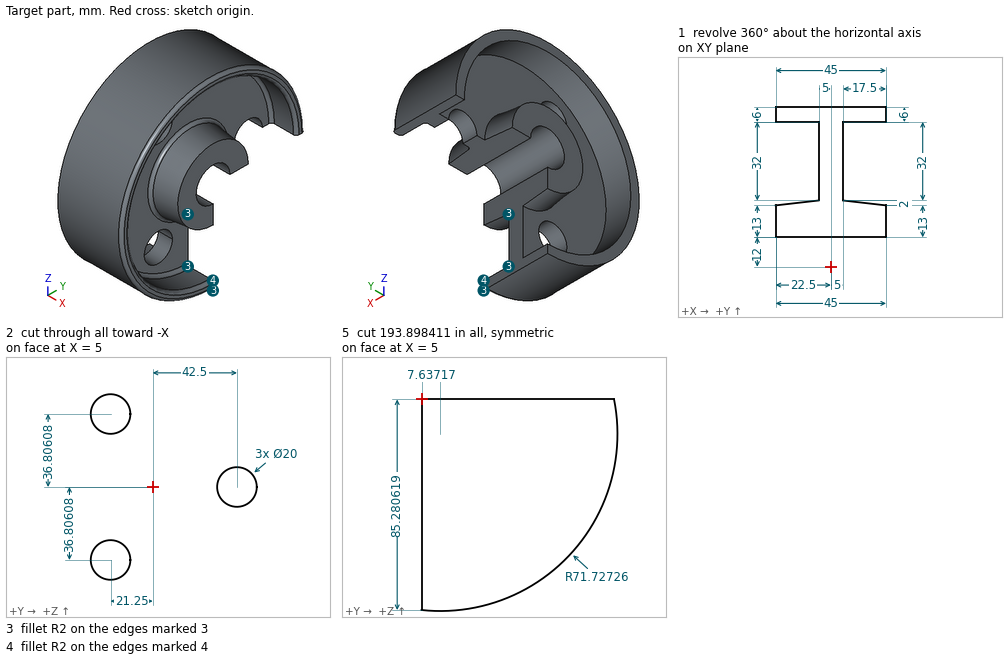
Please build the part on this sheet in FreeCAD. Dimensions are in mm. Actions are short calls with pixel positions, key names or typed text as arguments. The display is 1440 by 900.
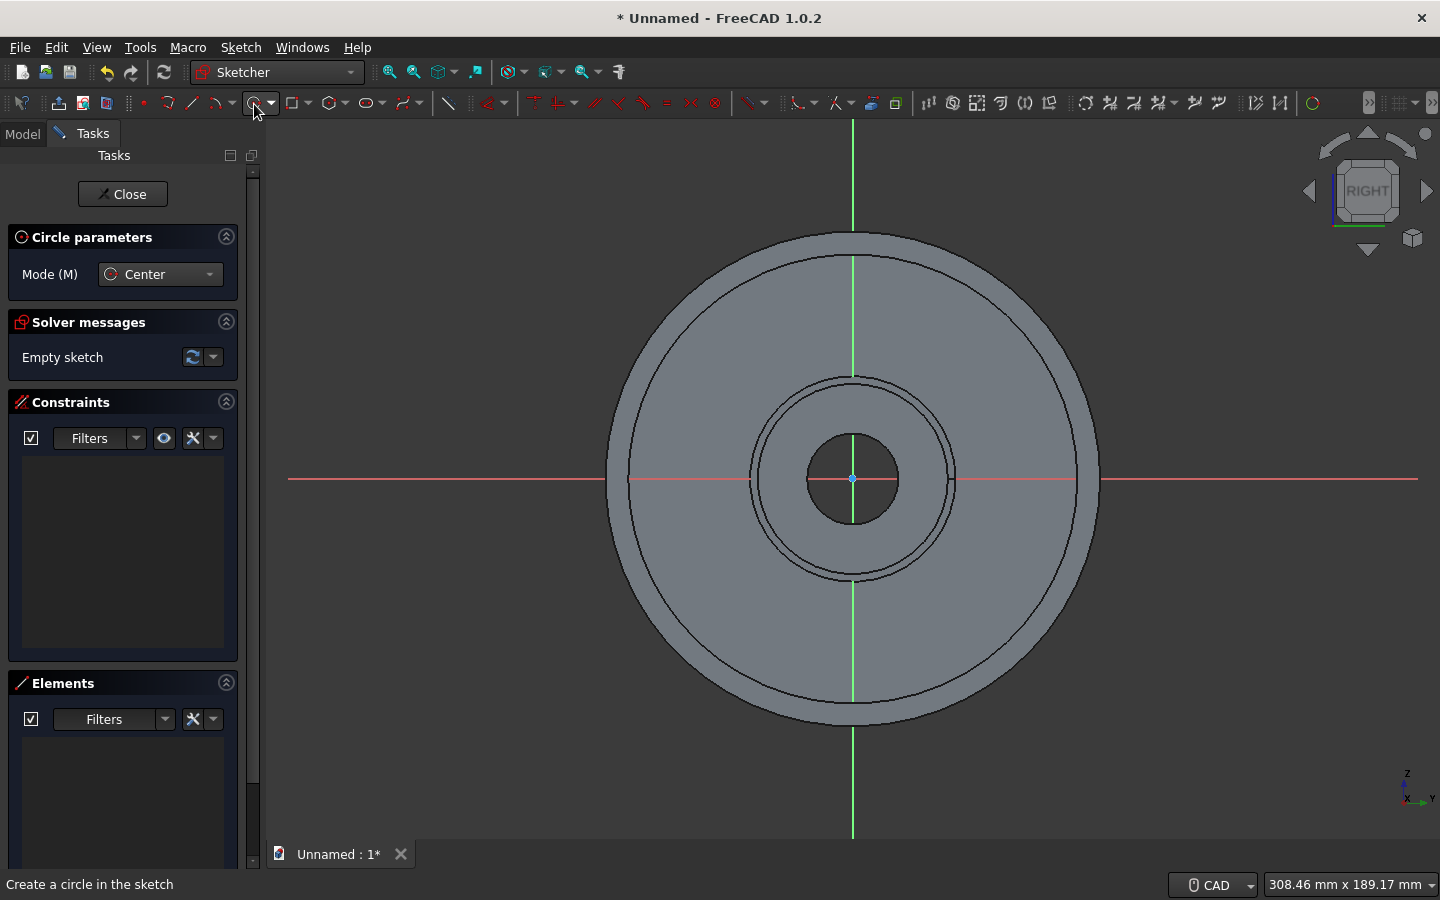
click(1015, 479)
move(1041, 452)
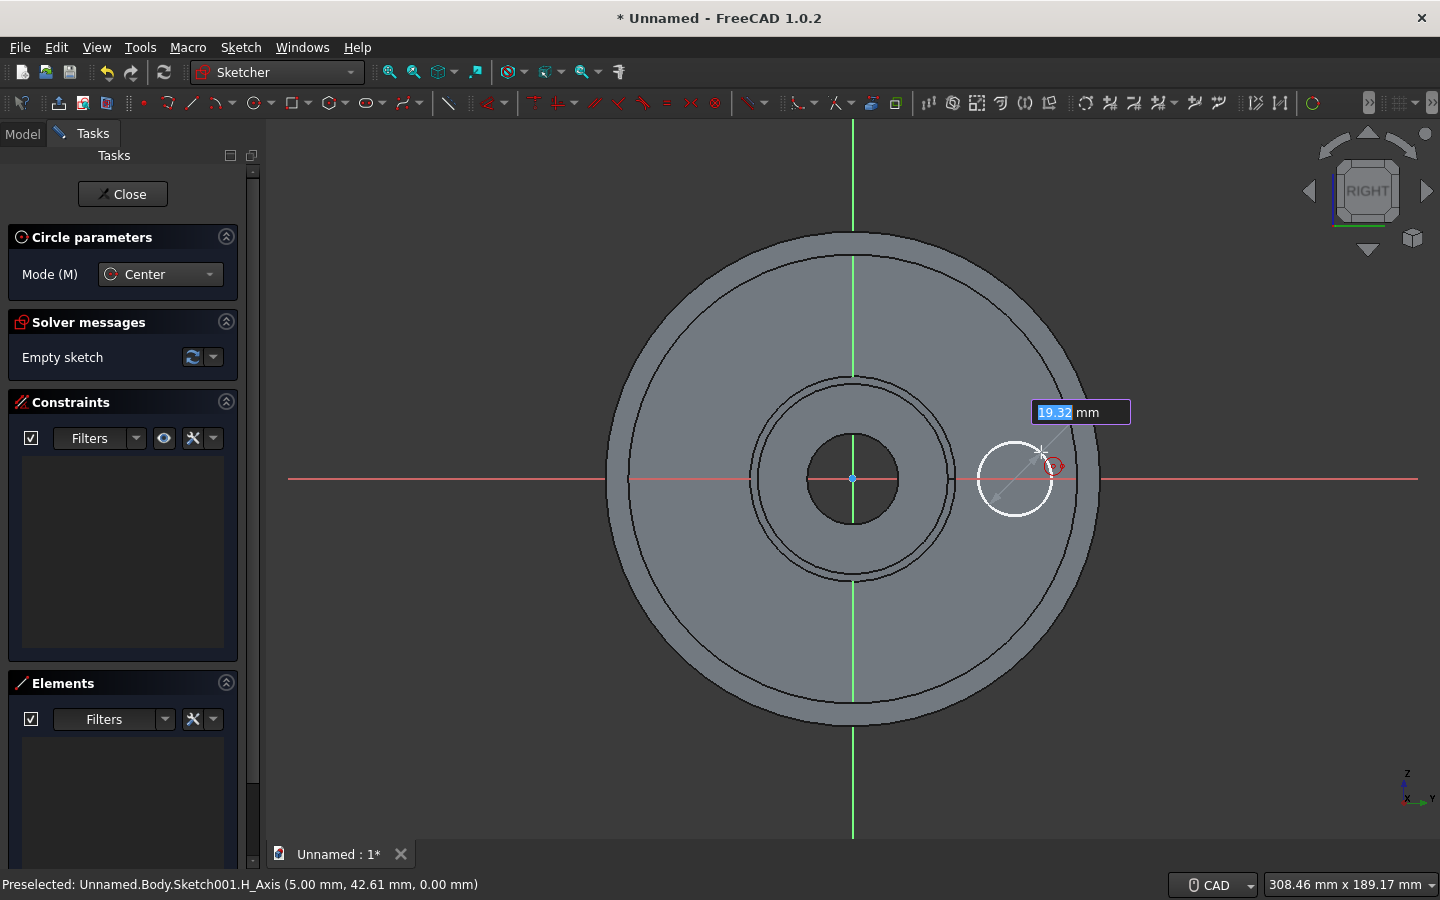
text(20)
key(Return)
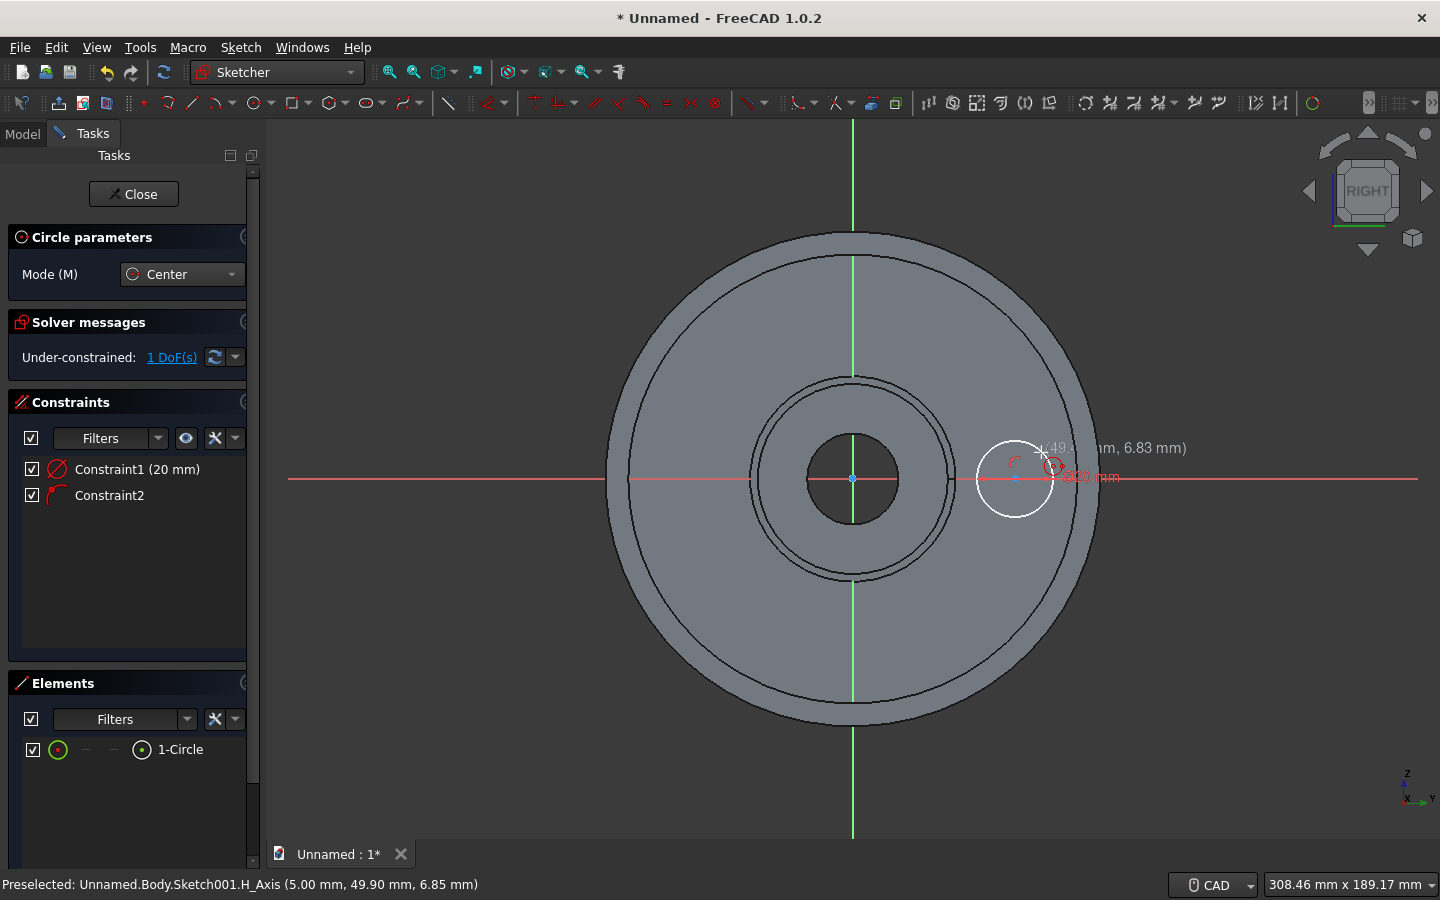
click(772, 619)
move(799, 592)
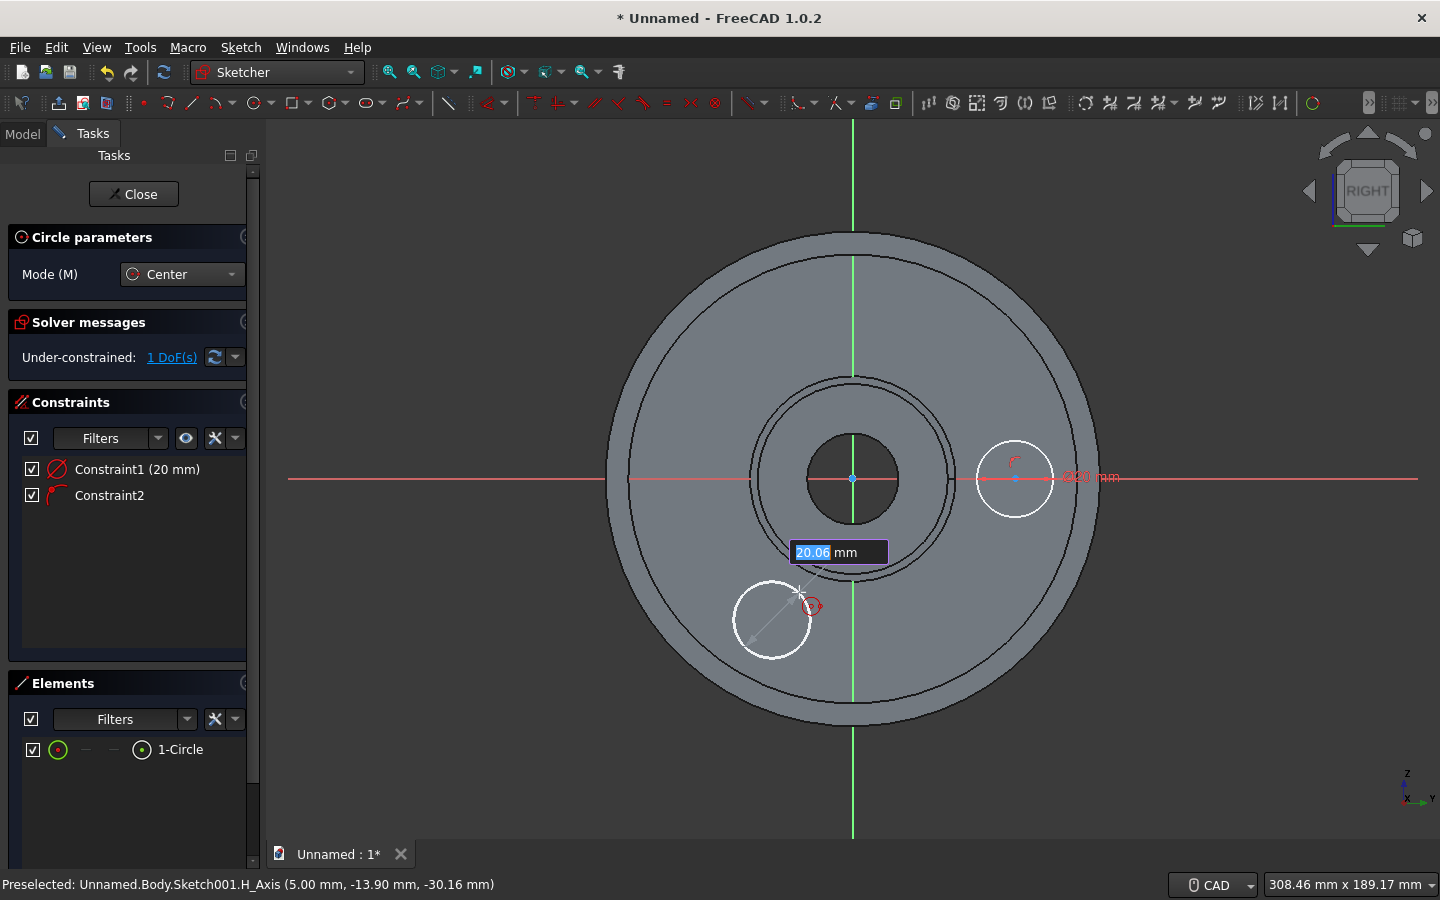
text(20)
key(Return)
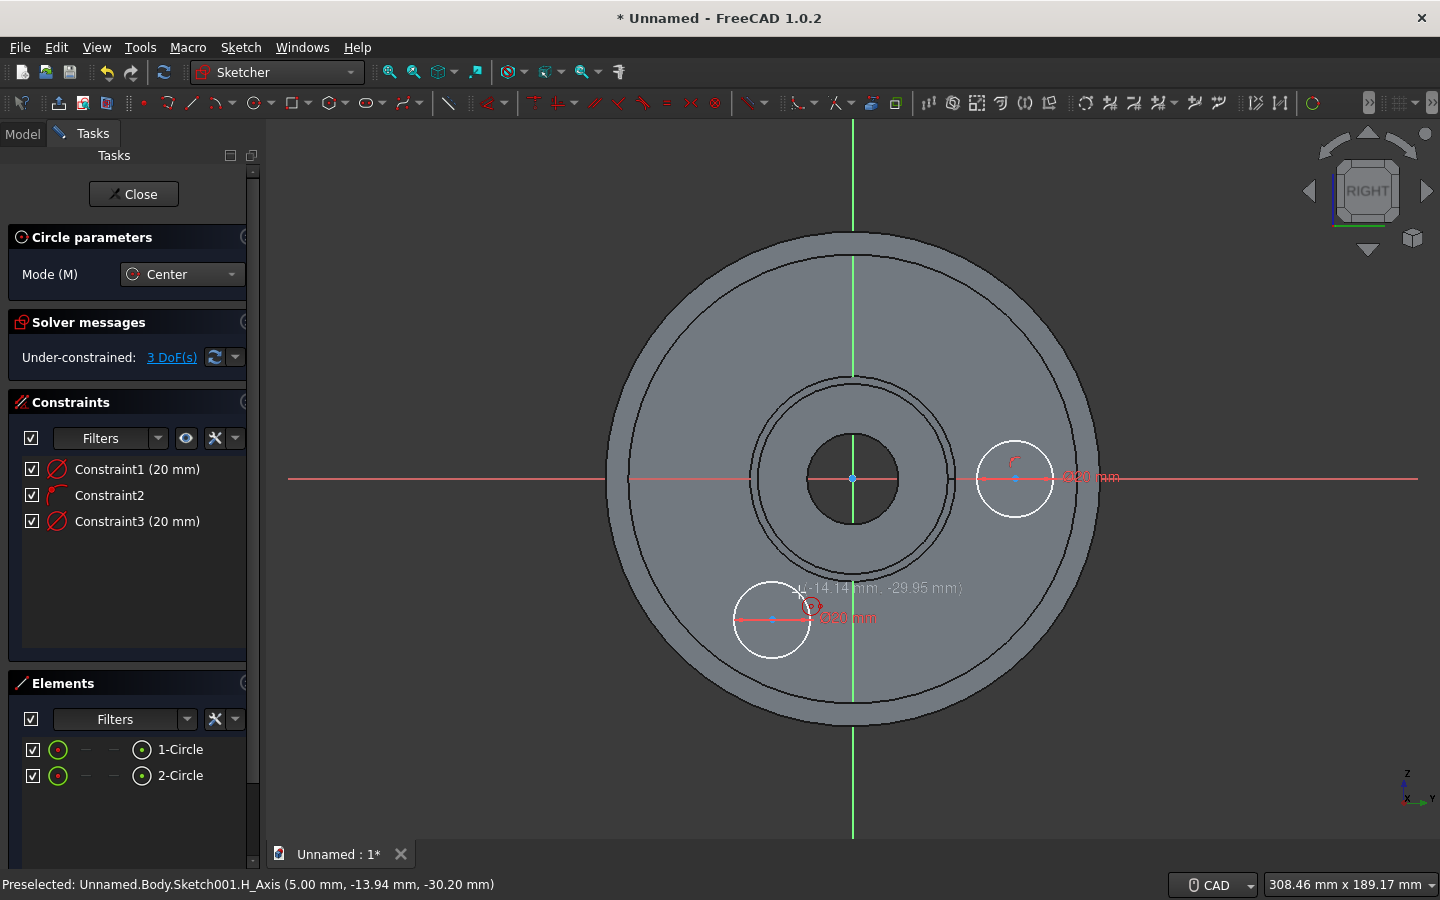
click(772, 339)
move(799, 312)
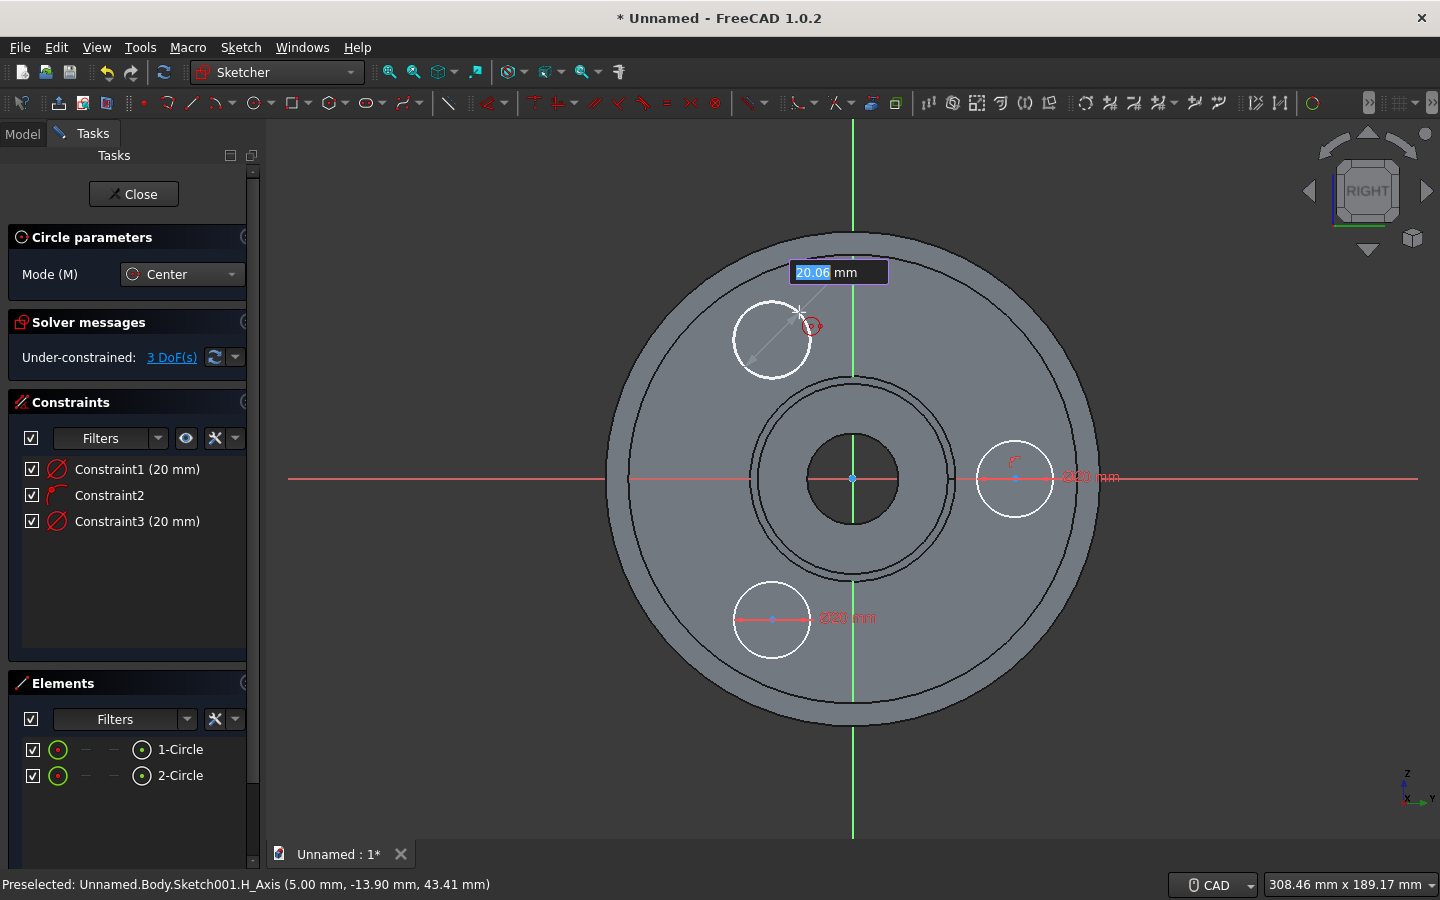
text(20)
key(Return)
key(Escape)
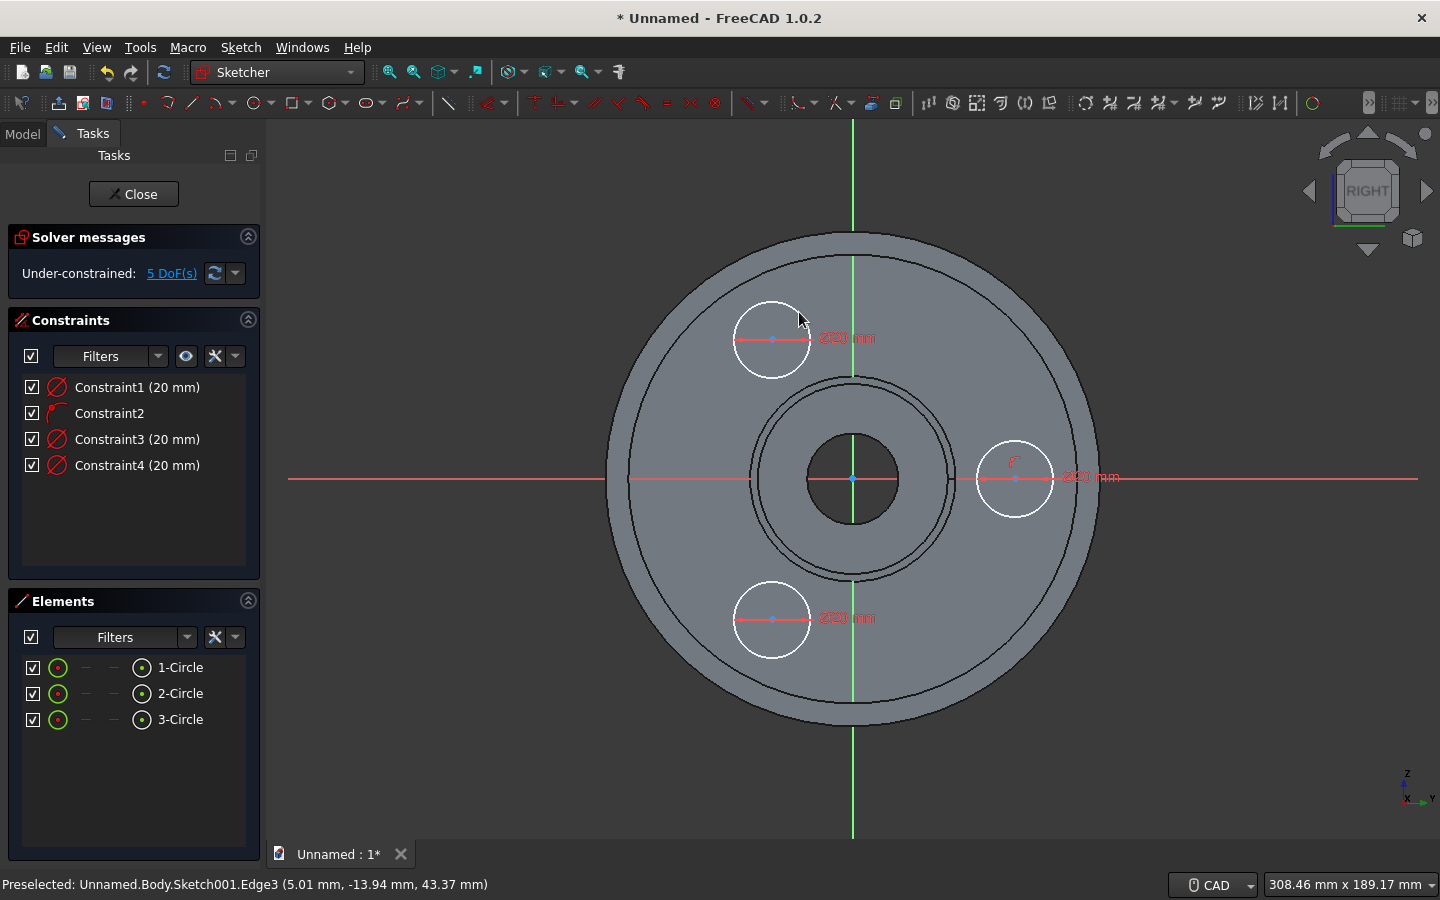
click(772, 620)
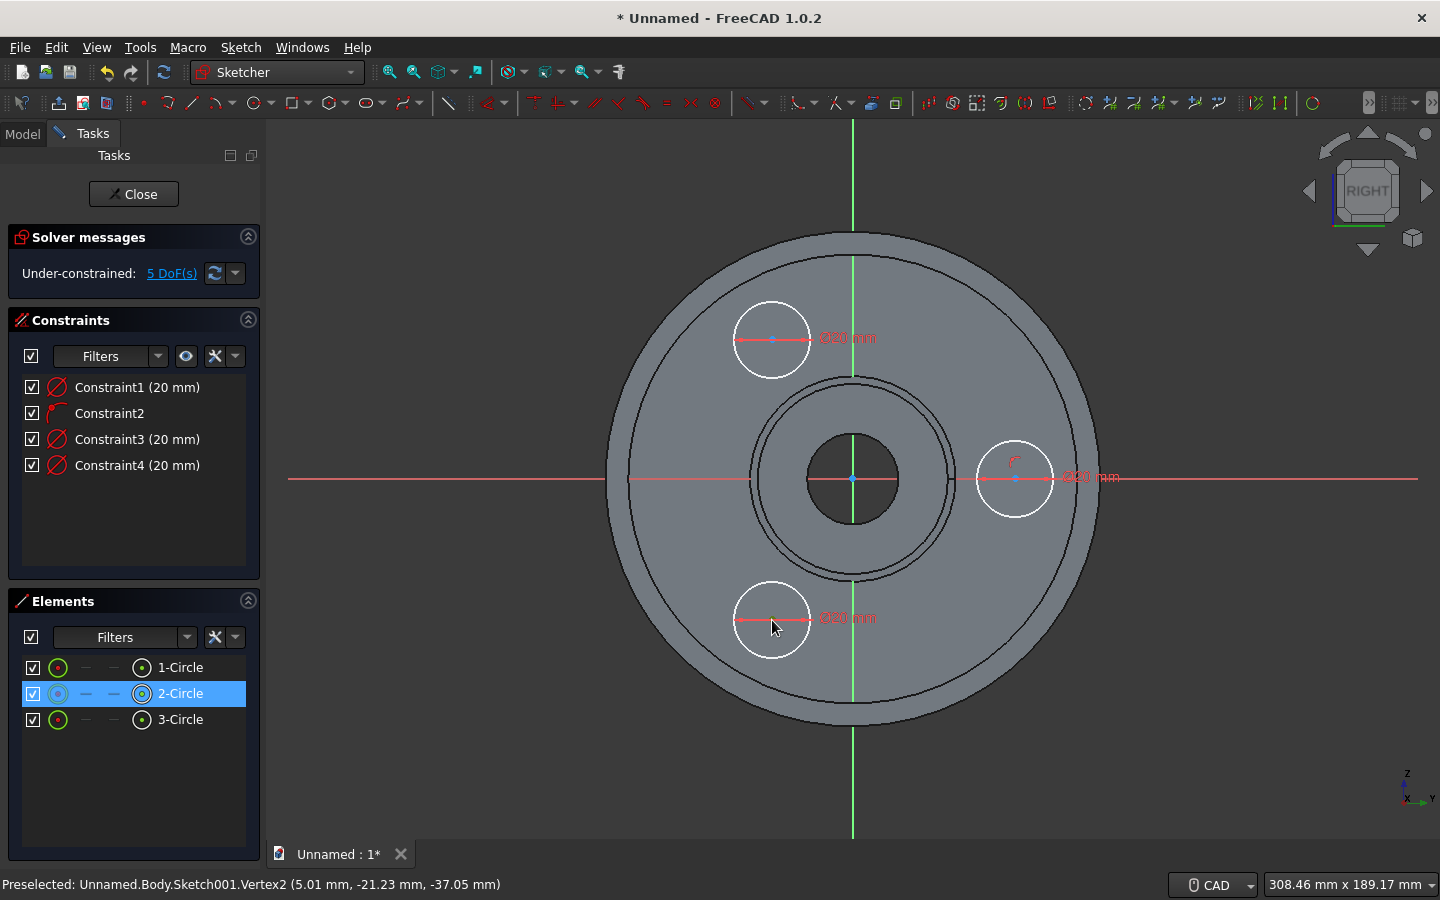
click(772, 340)